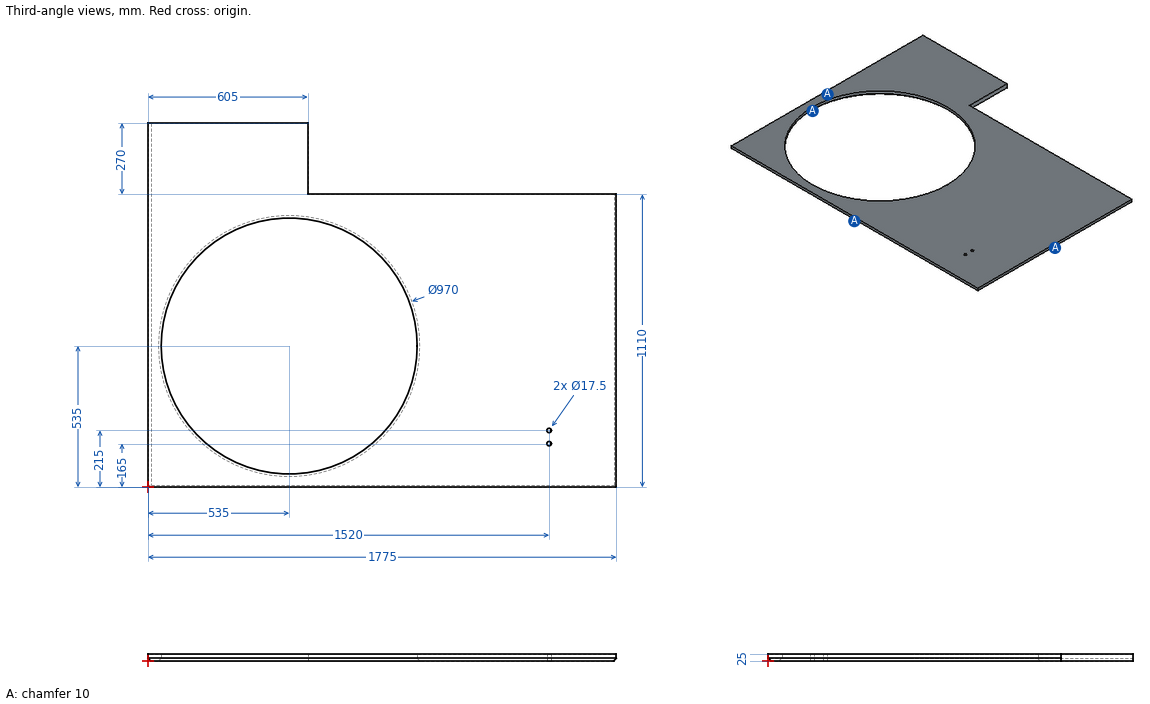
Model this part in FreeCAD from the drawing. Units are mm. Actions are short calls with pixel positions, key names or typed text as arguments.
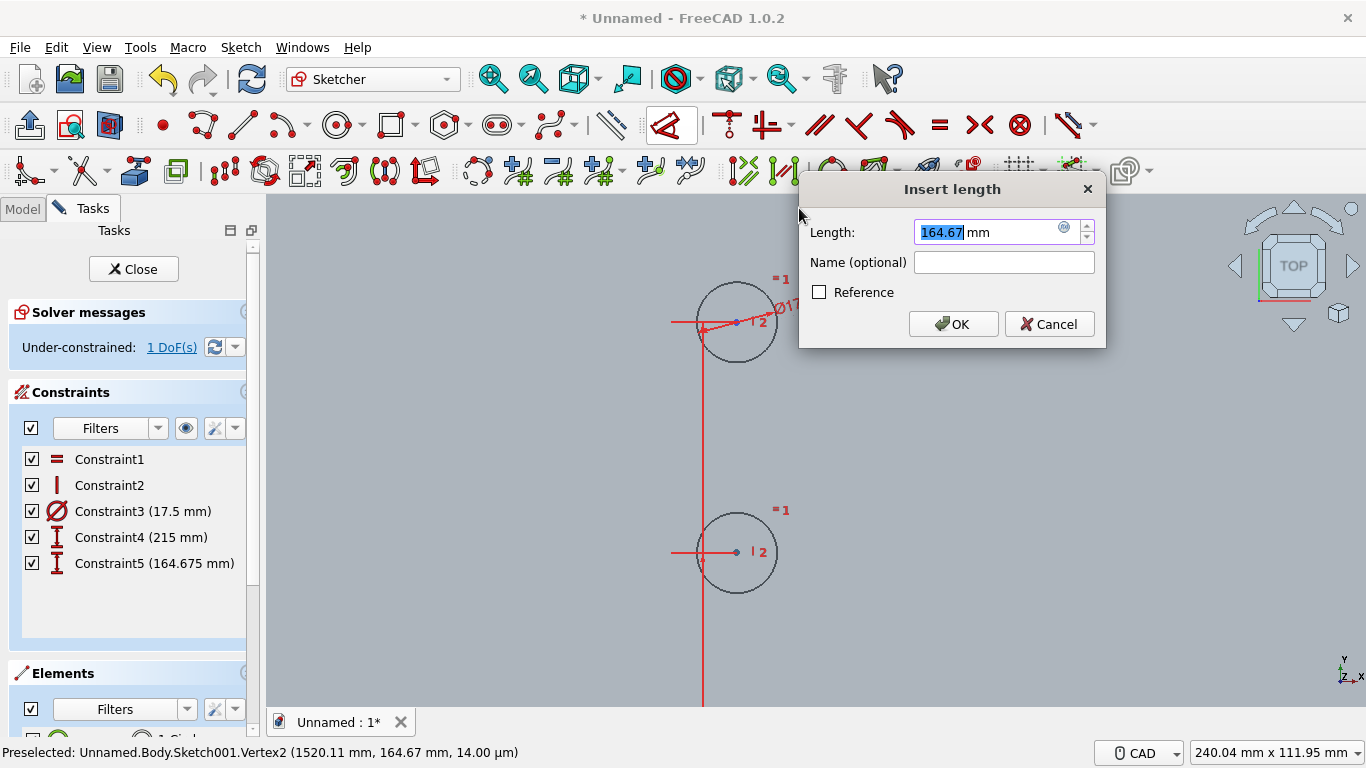
text(165)
key(Return)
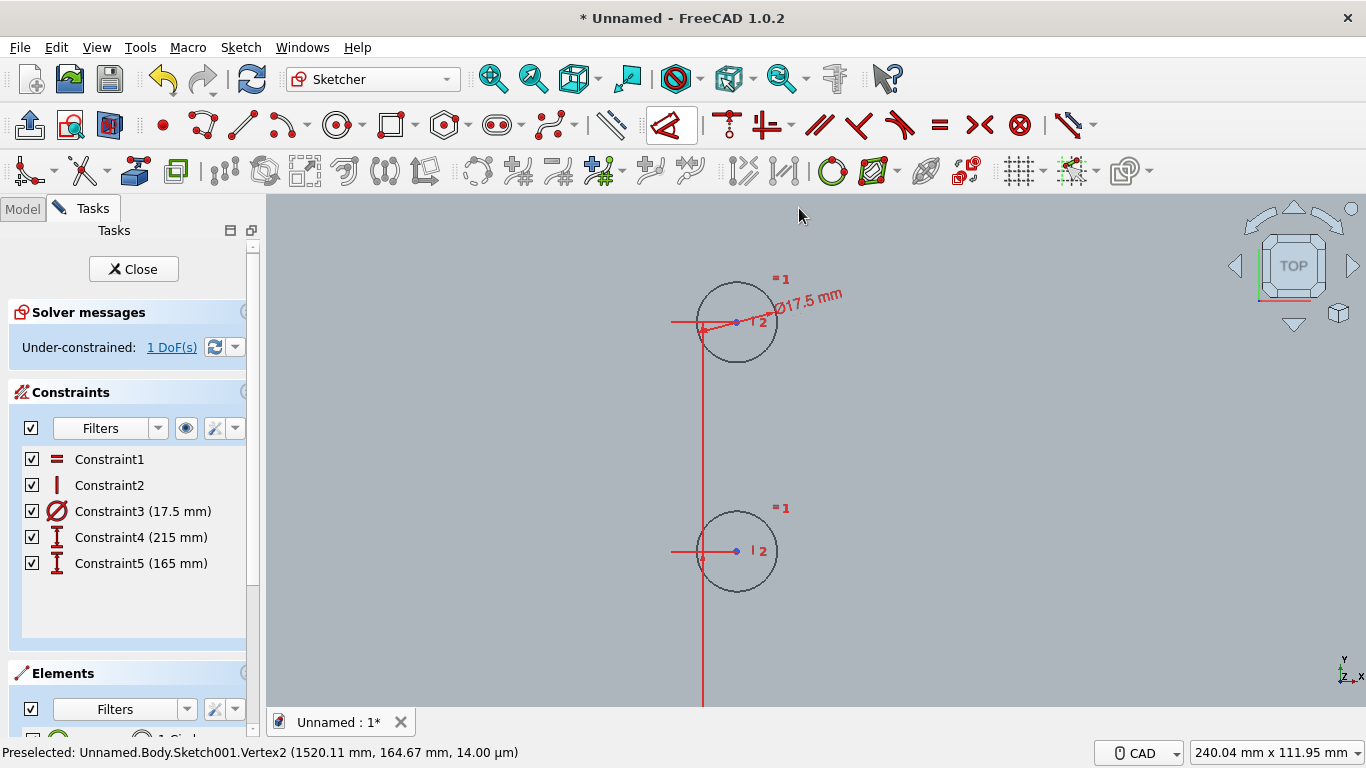
click(737, 322)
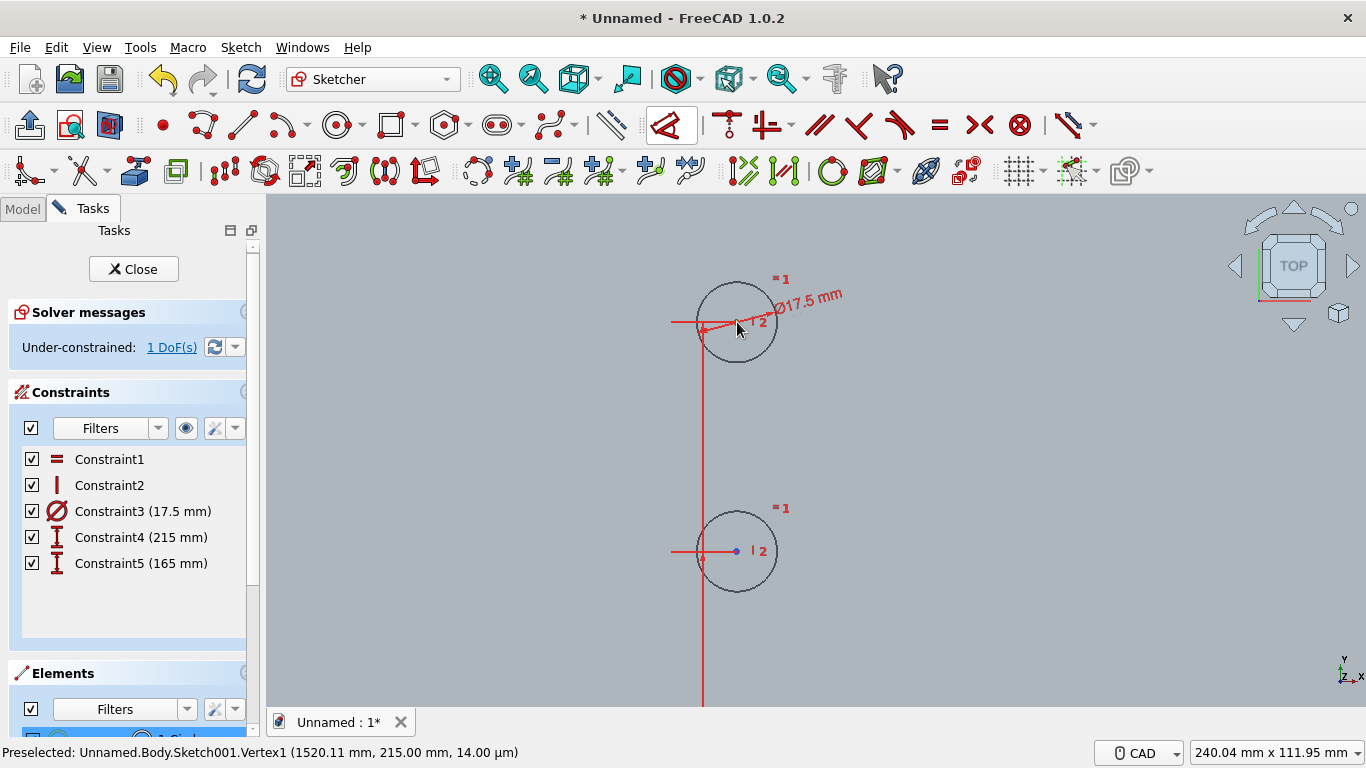
click(692, 126)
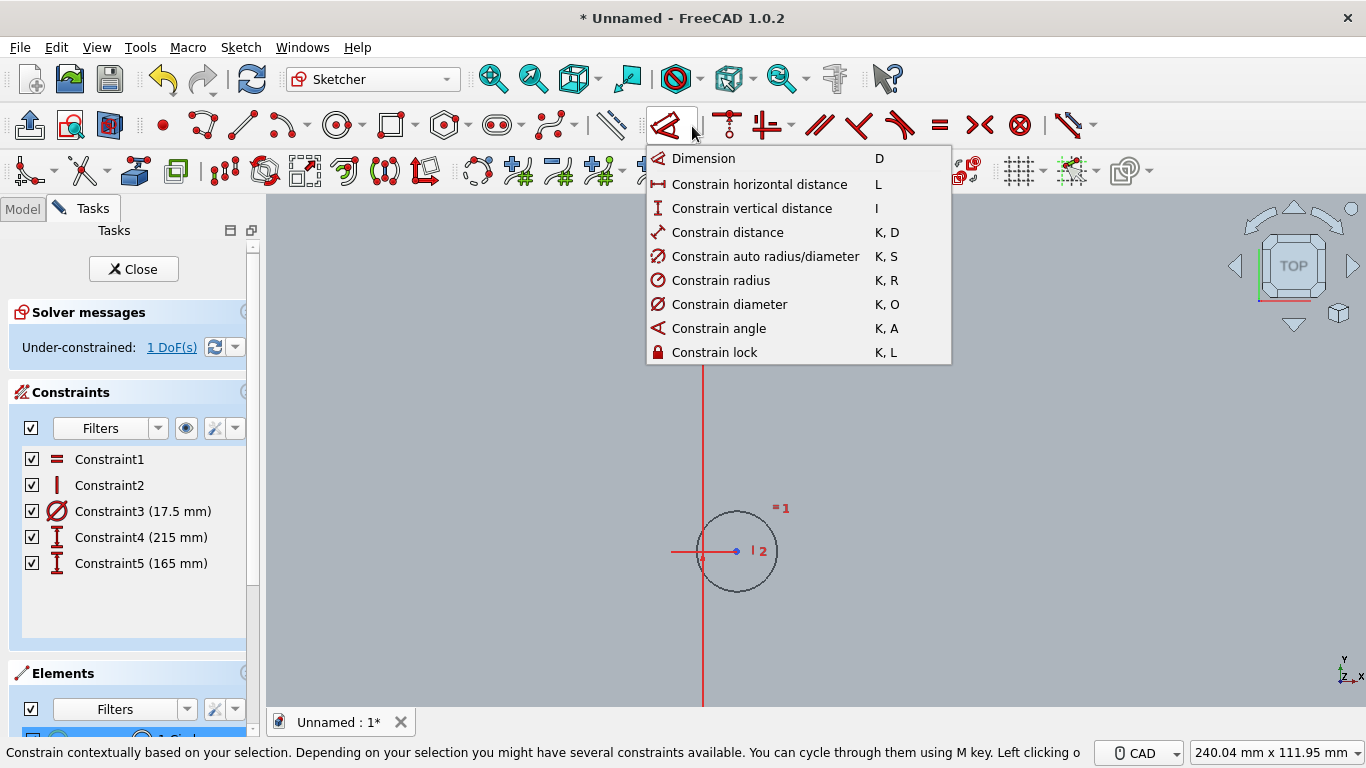
click(799, 184)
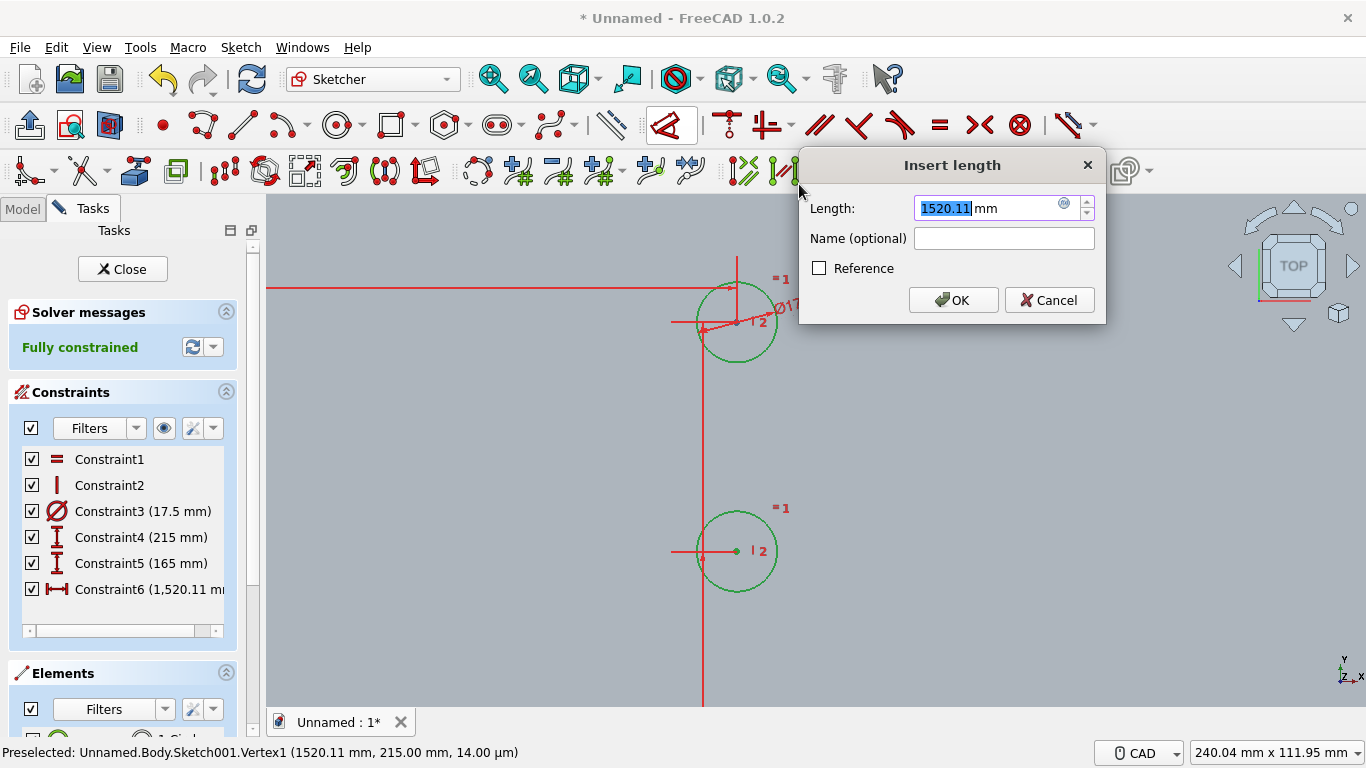
text(1520)
key(Return)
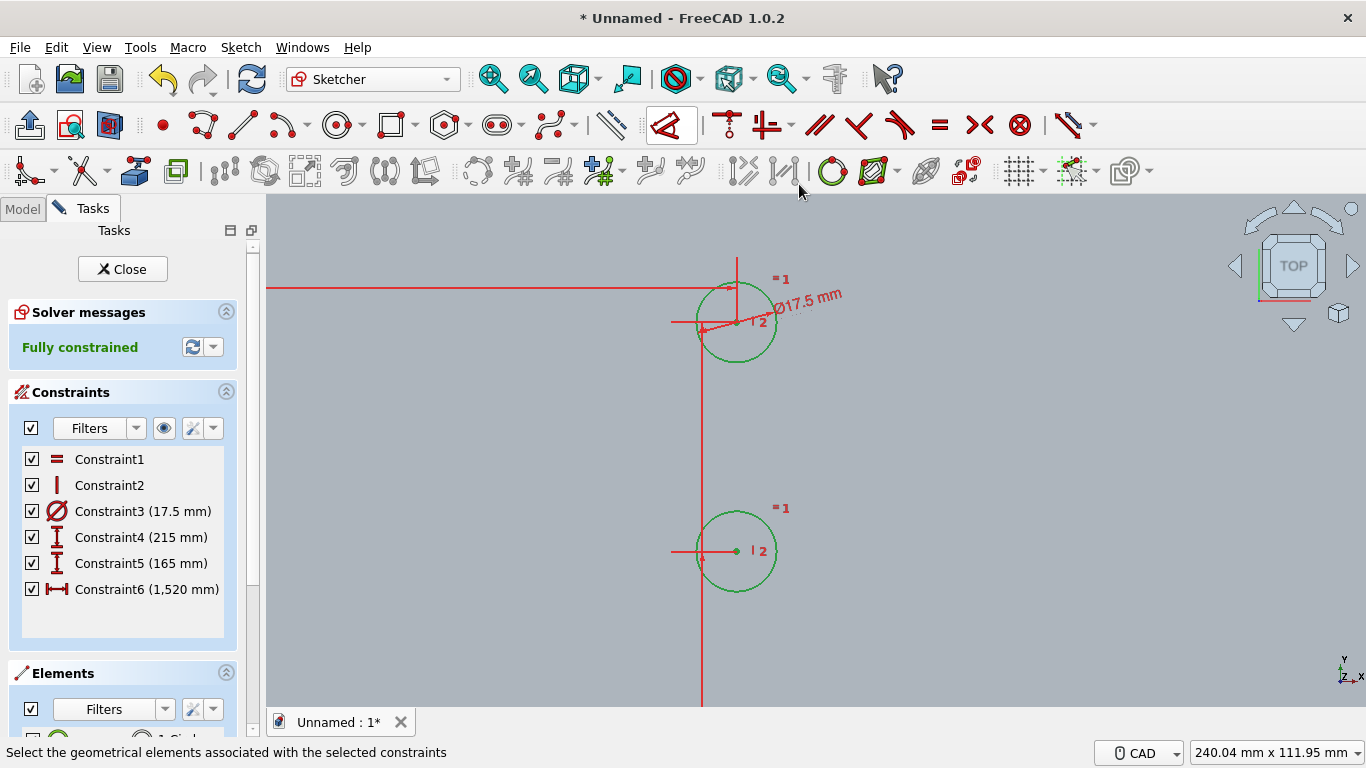
click(123, 269)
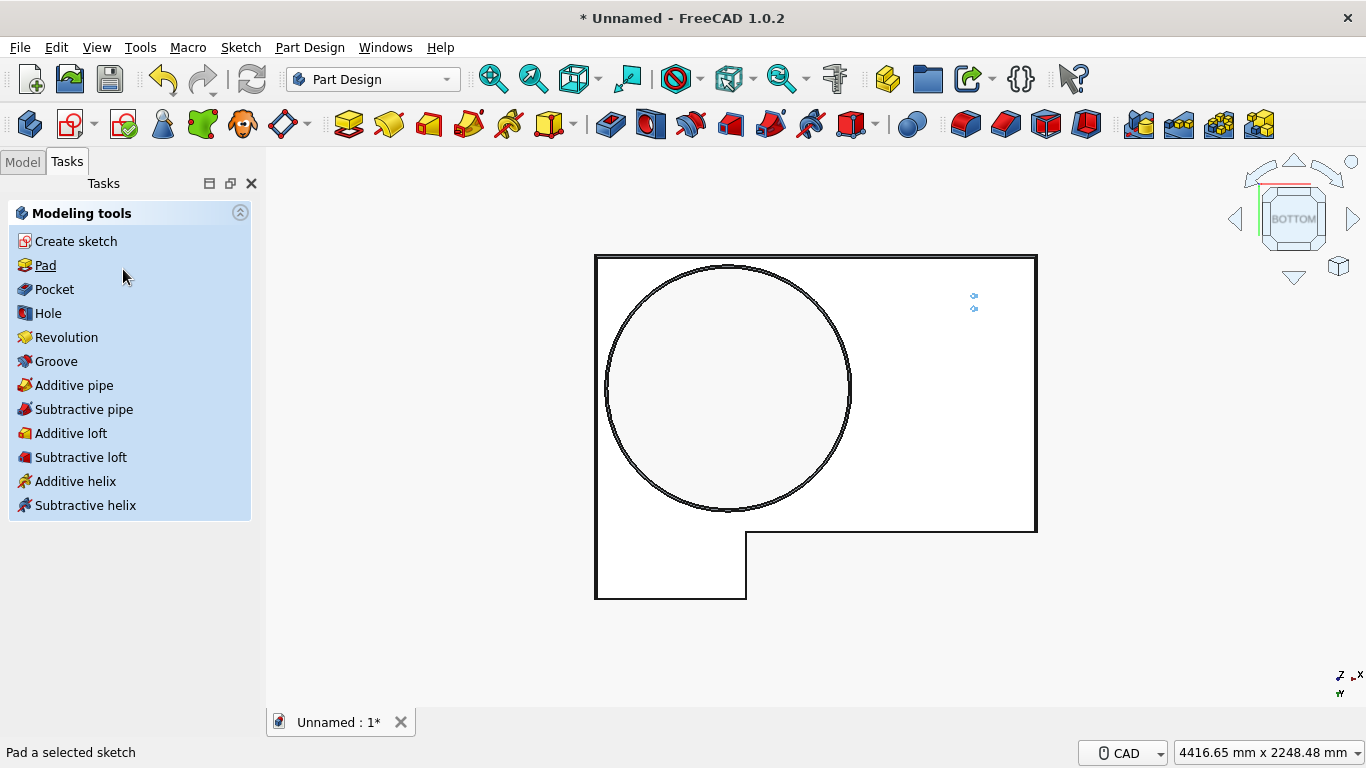
click(612, 124)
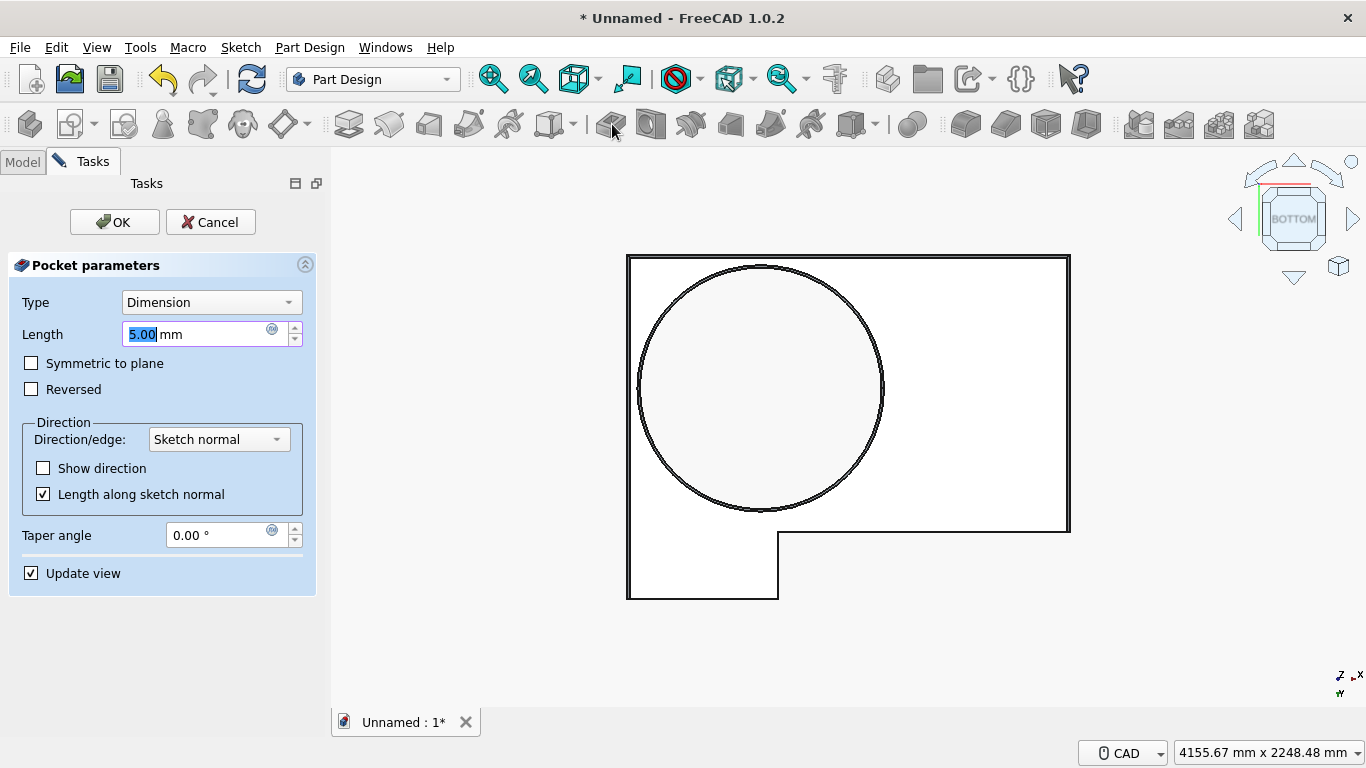
click(212, 302)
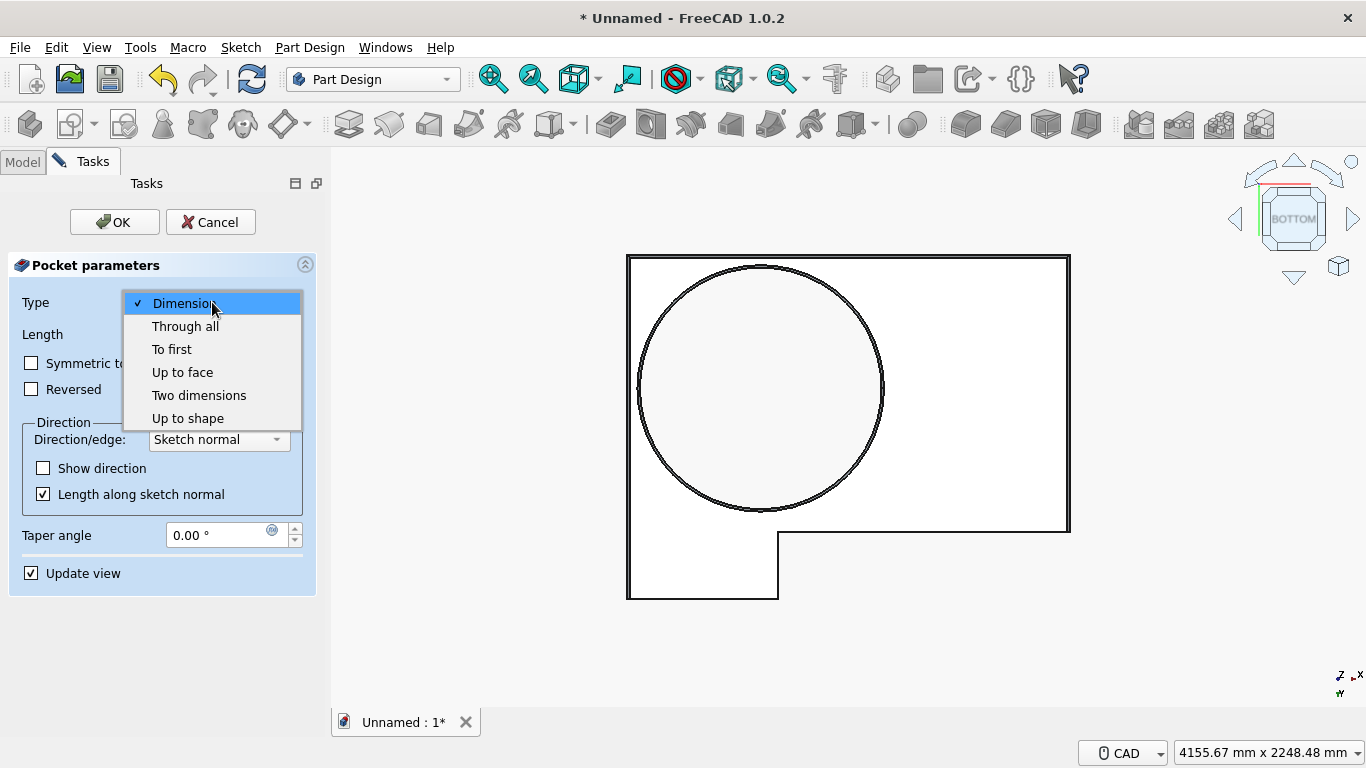
click(212, 326)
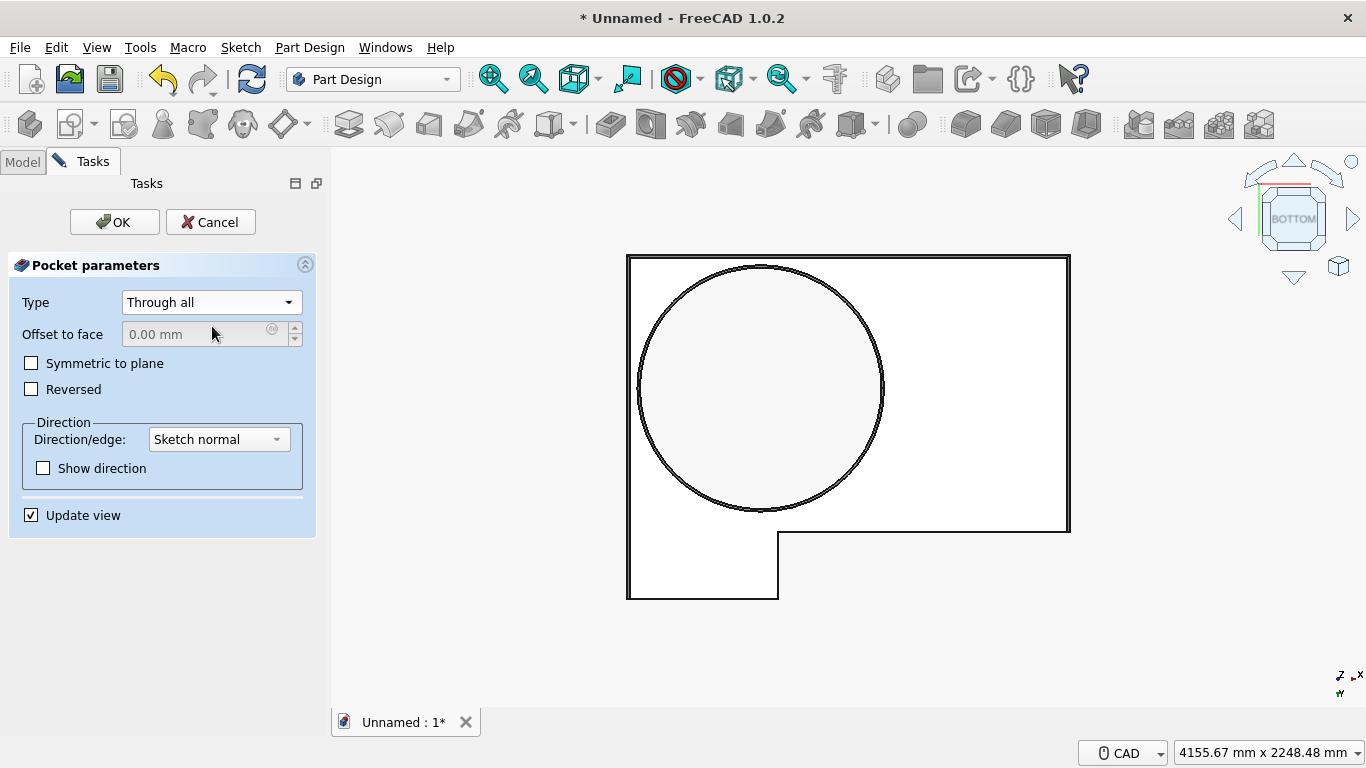
click(30, 389)